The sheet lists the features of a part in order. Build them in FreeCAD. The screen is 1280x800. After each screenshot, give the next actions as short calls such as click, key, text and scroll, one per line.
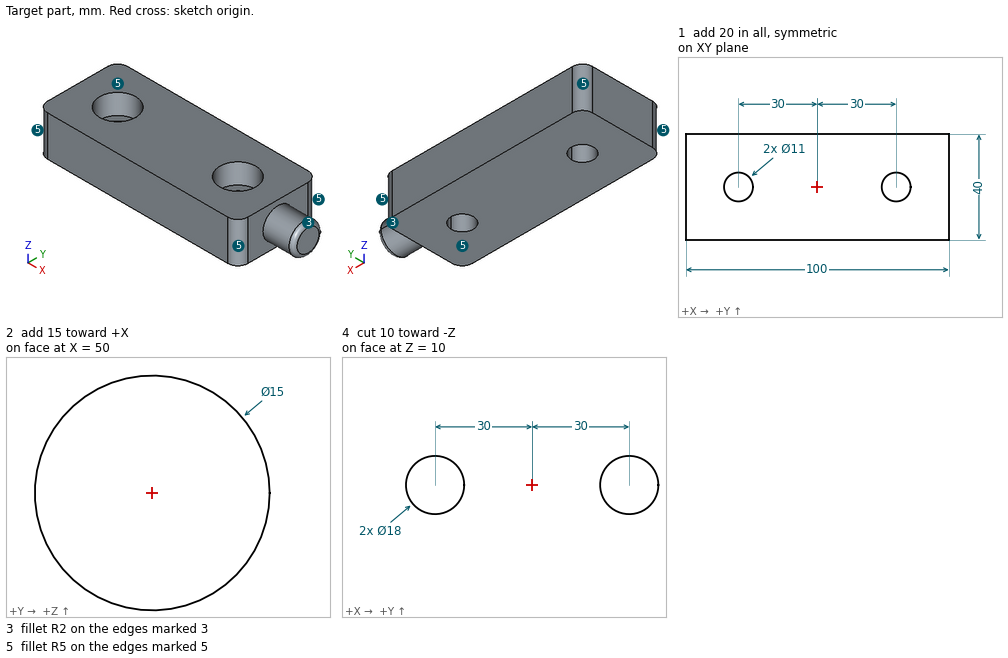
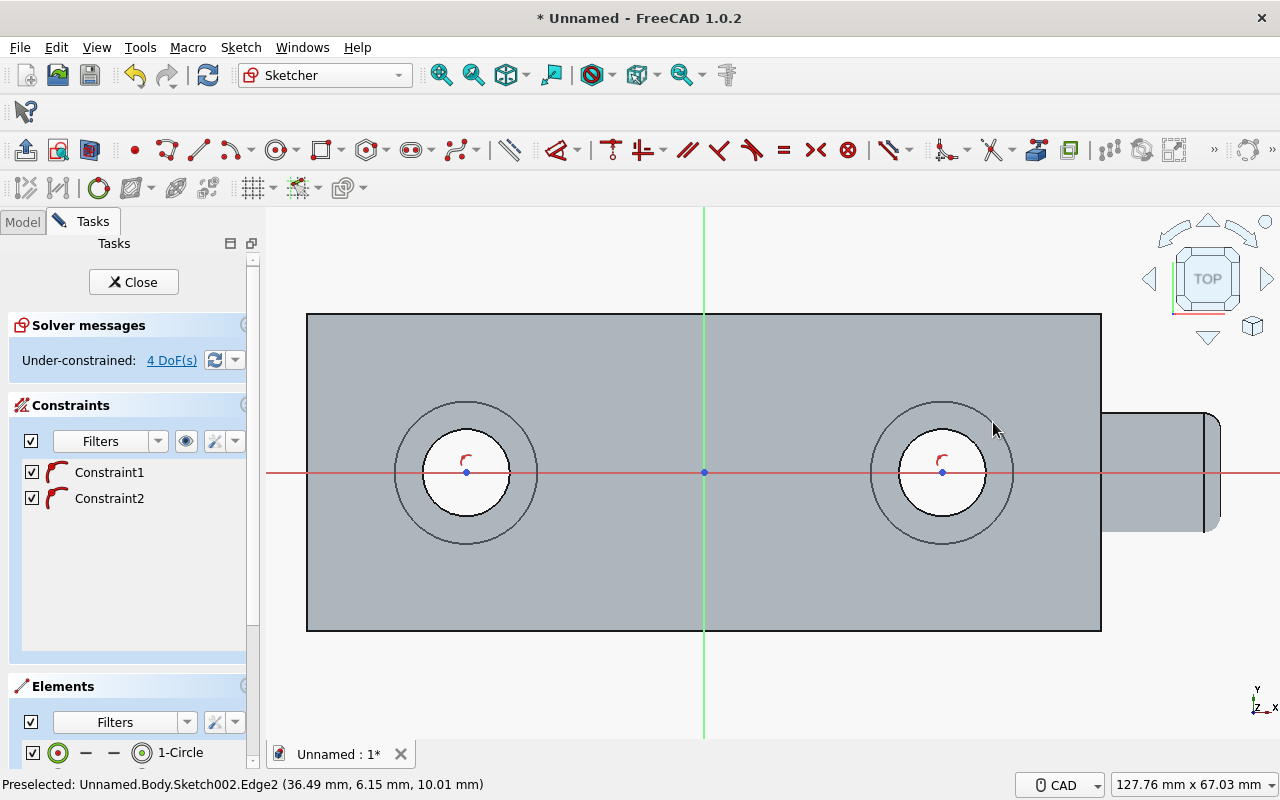
click(516, 422)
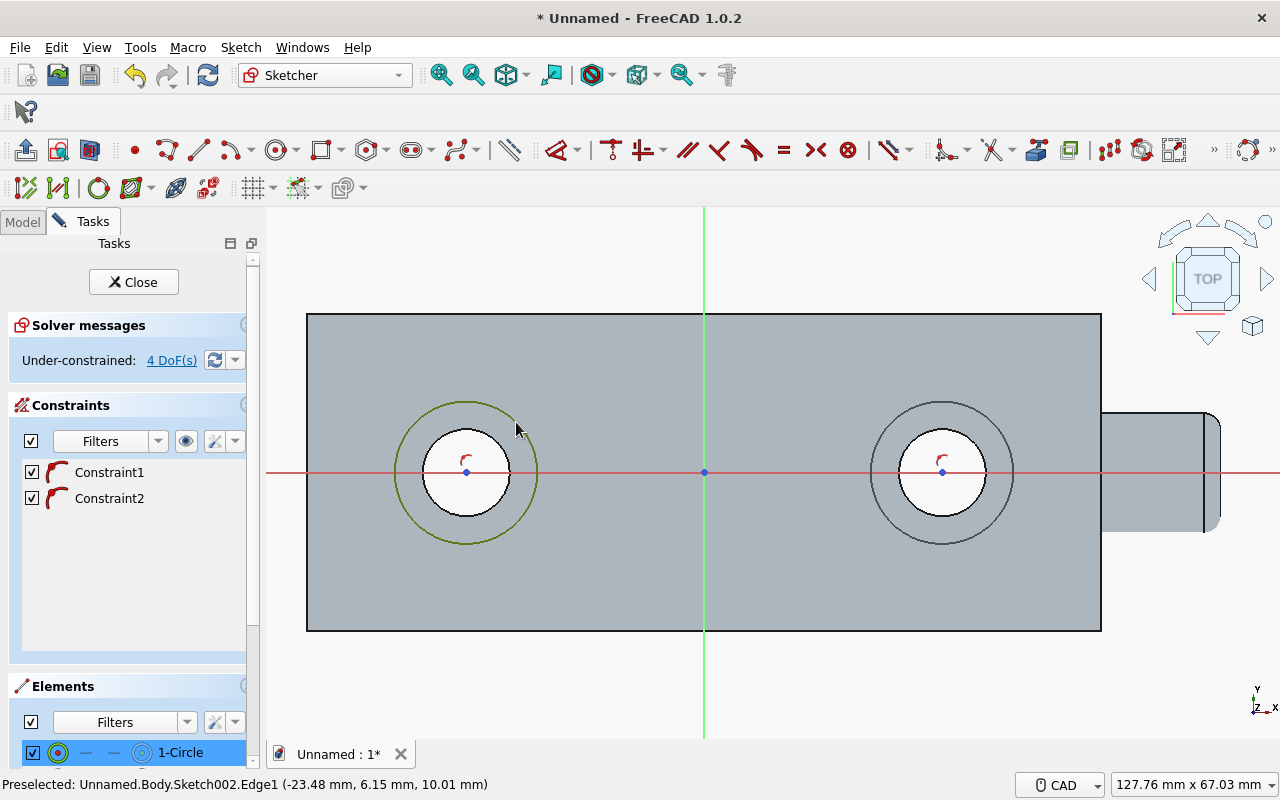
click(992, 422)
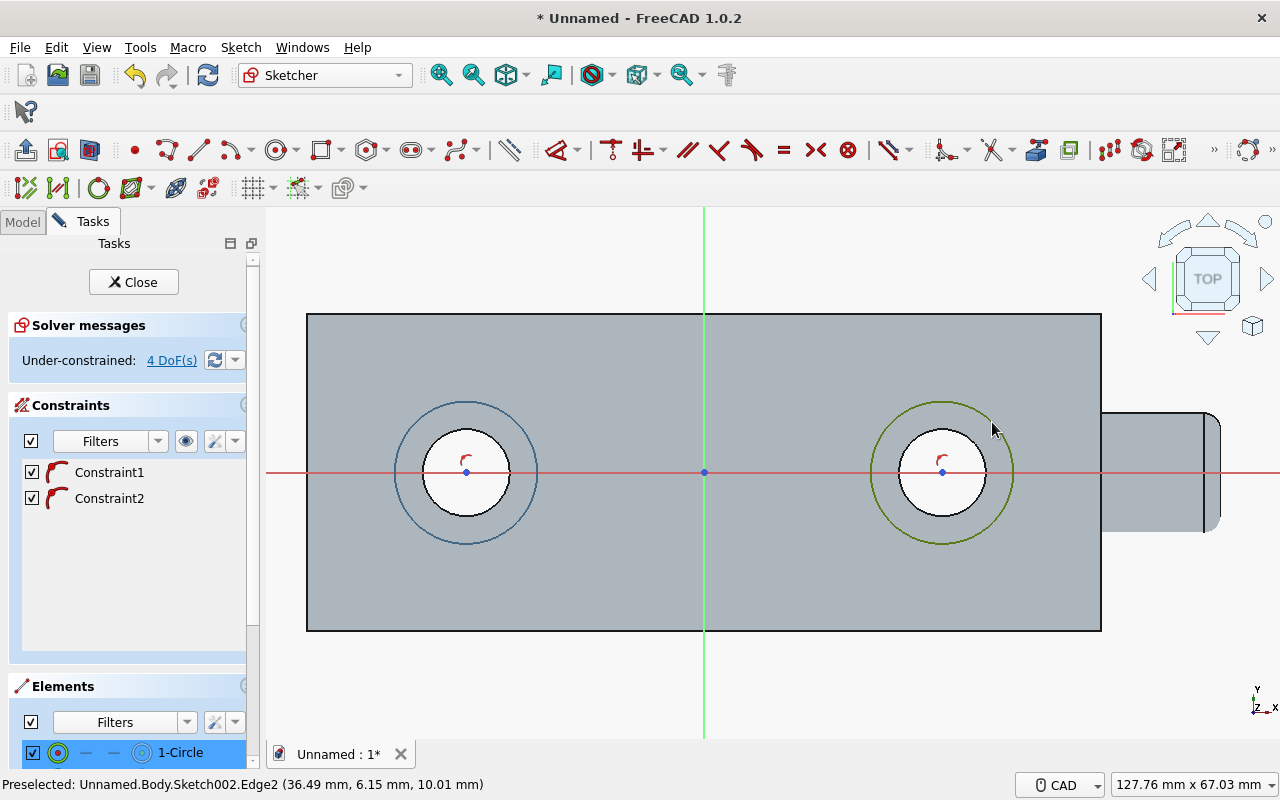
click(784, 150)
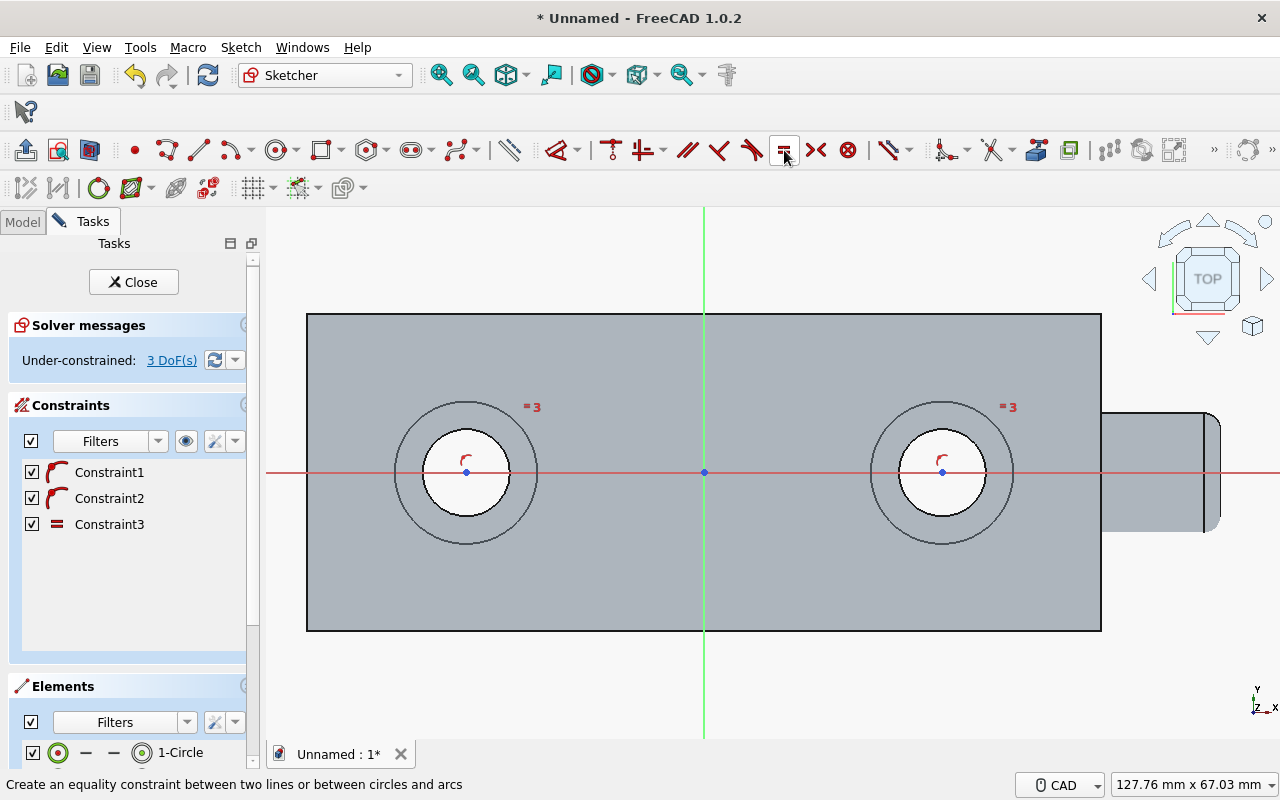
click(556, 150)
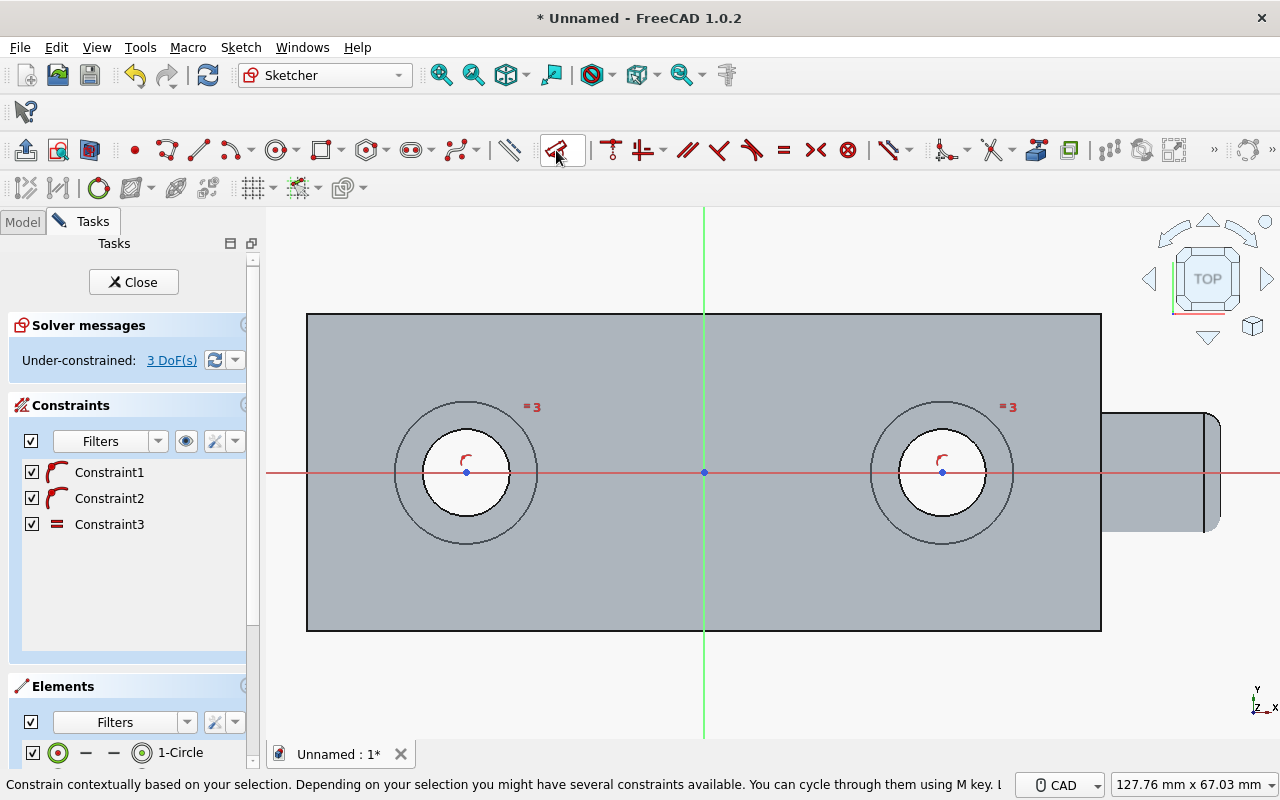
click(516, 422)
click(538, 399)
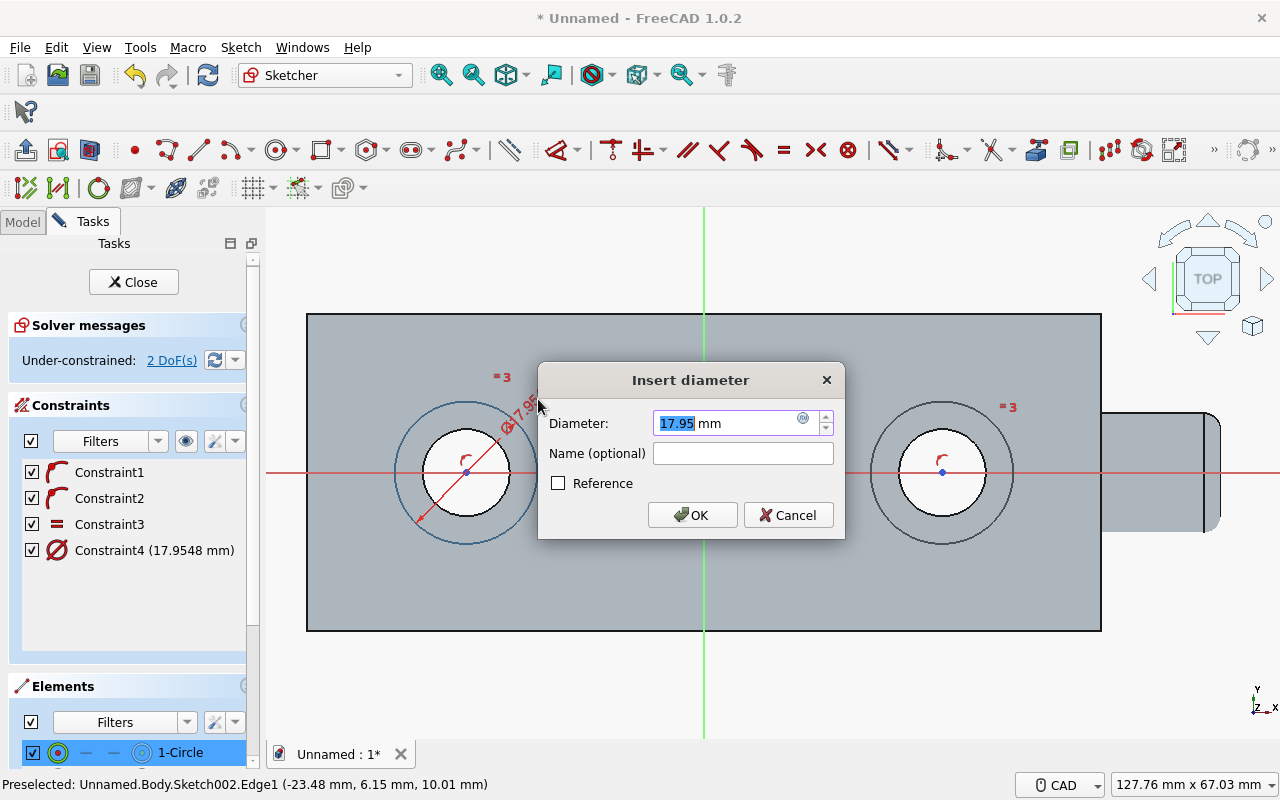
text(18)
key(Return)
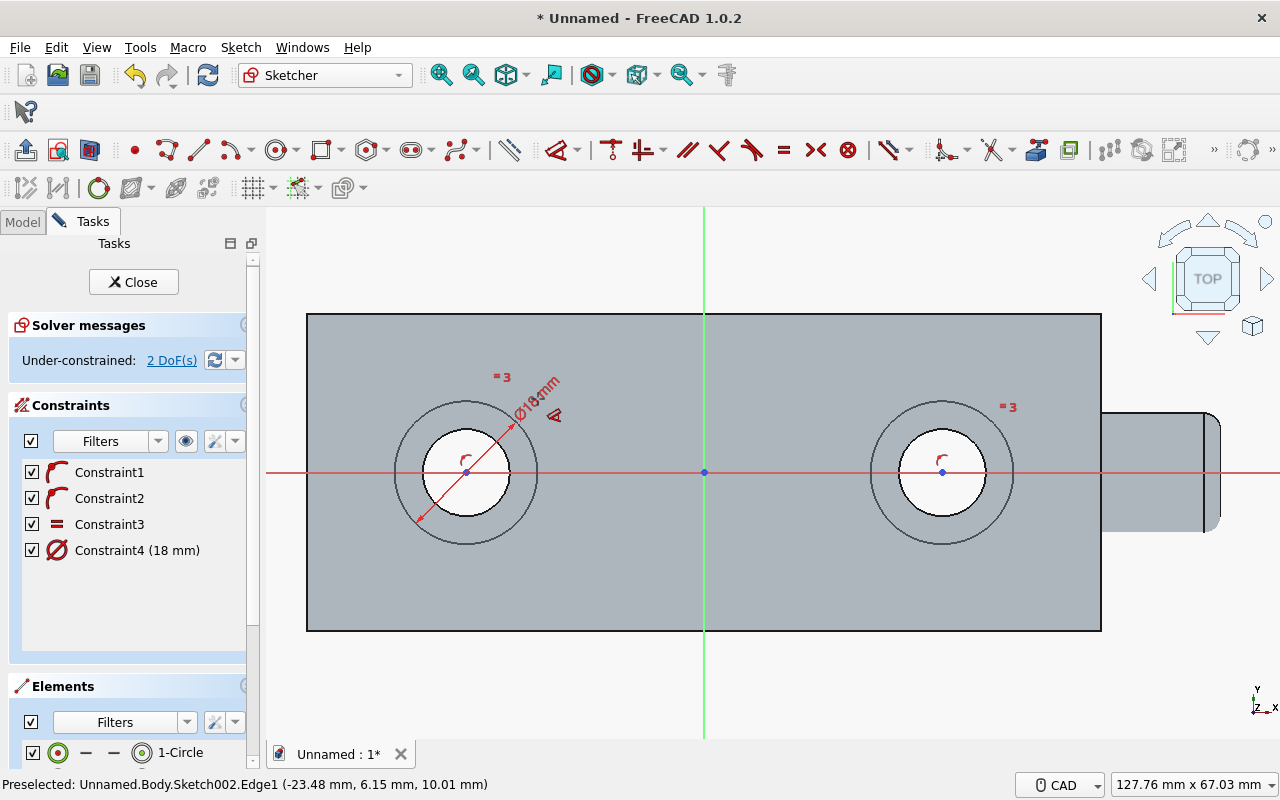
click(466, 473)
click(585, 507)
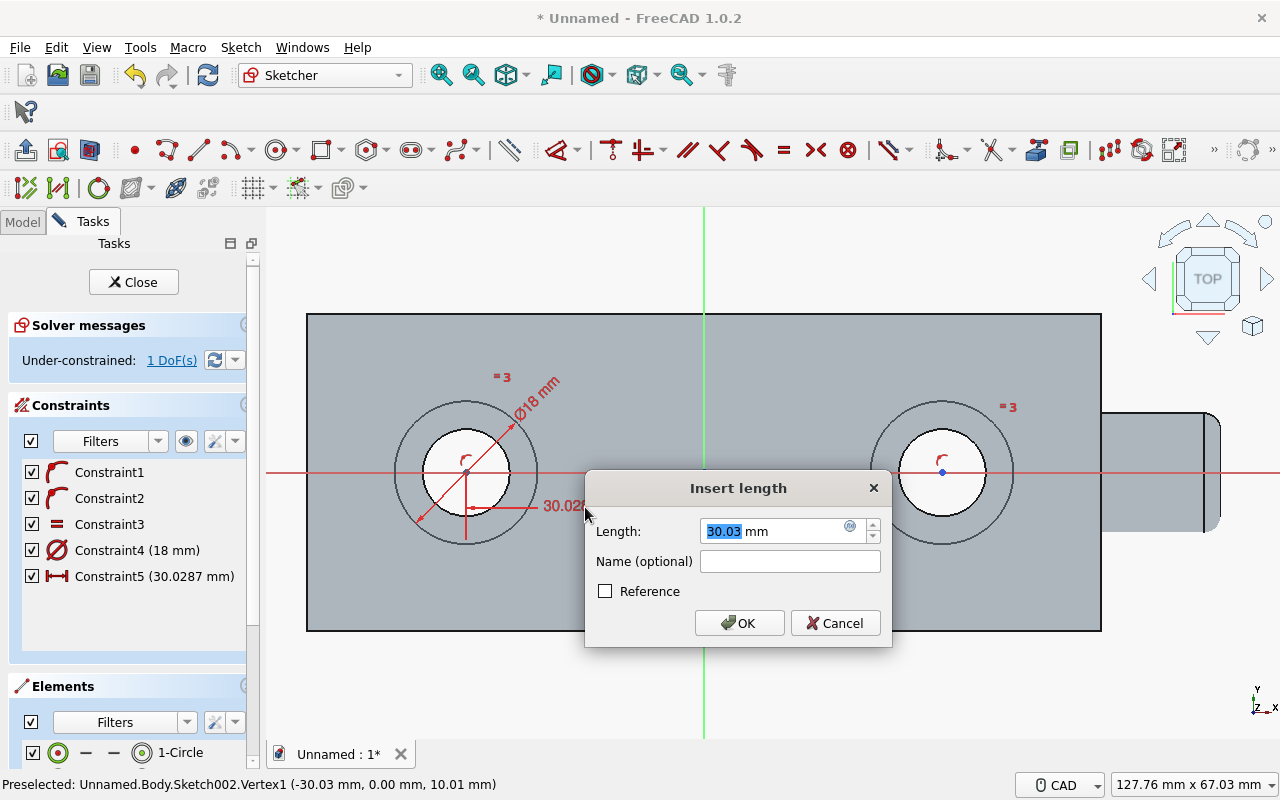
text(30)
key(Return)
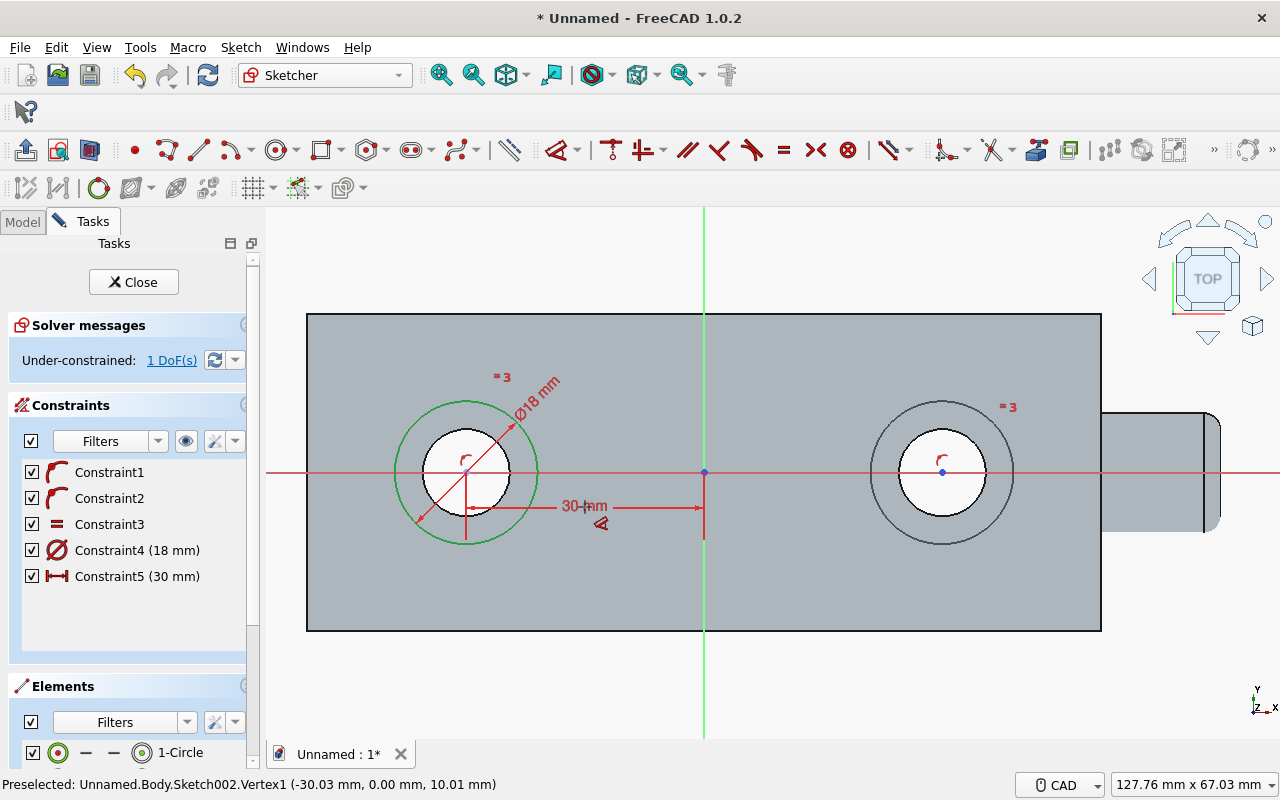
click(942, 473)
click(823, 507)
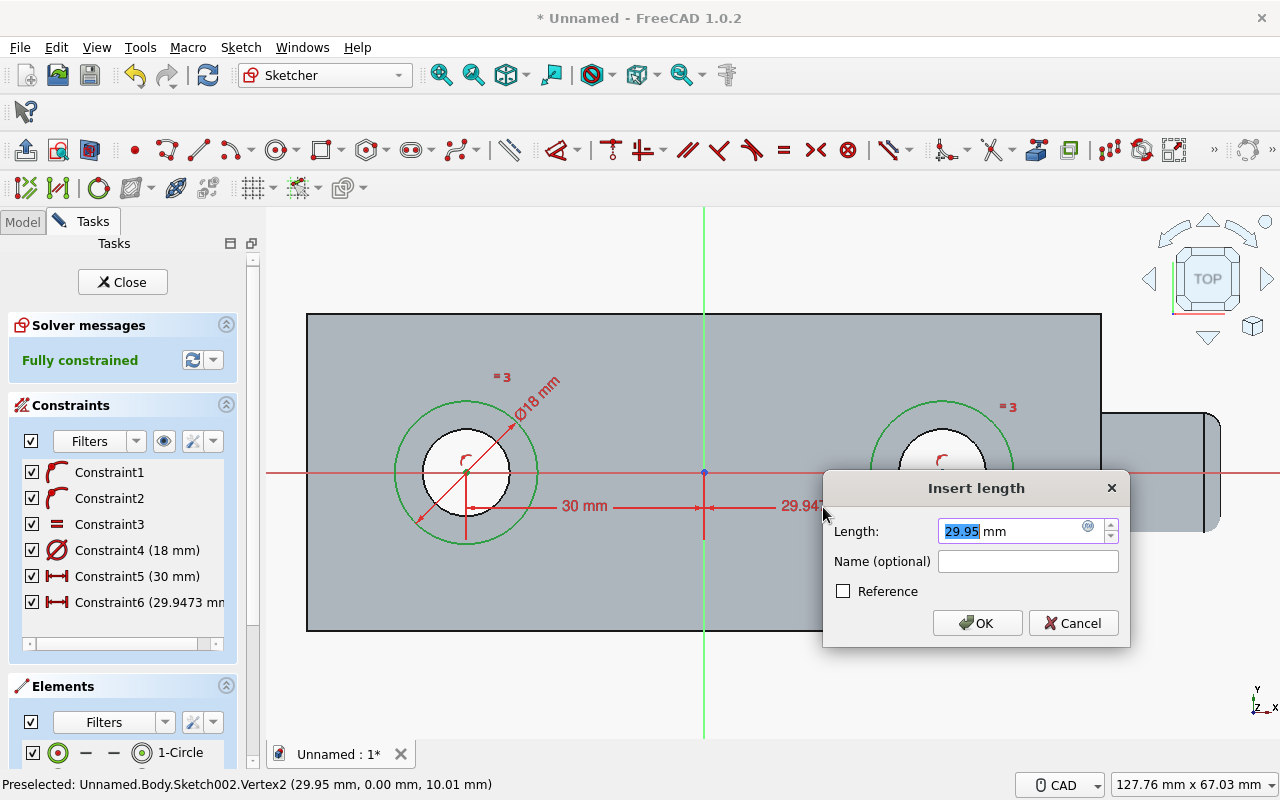
text(30)
key(Return)
key(Escape)